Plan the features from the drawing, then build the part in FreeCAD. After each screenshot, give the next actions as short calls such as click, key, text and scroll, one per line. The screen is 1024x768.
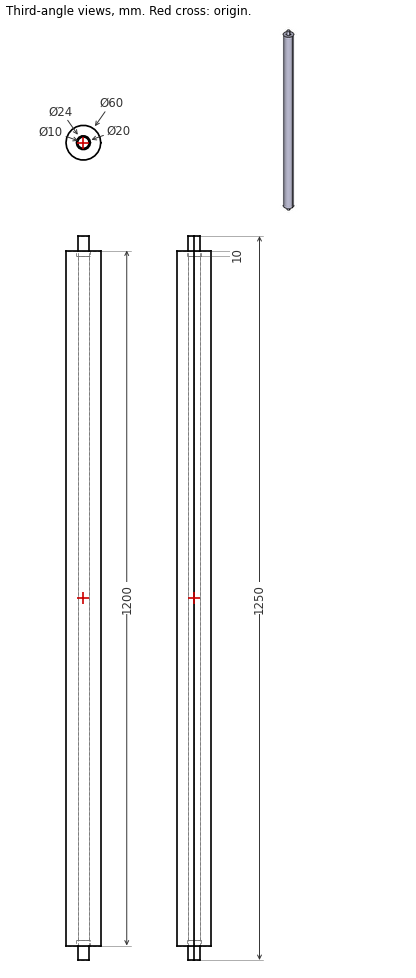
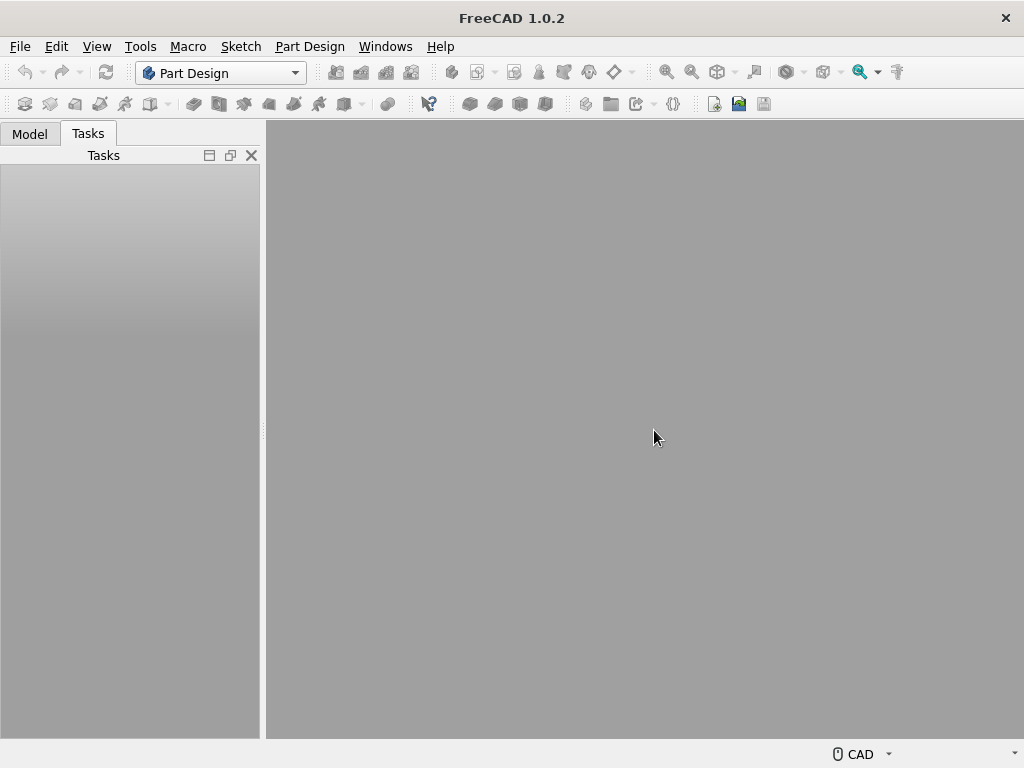
key(ctrl+n)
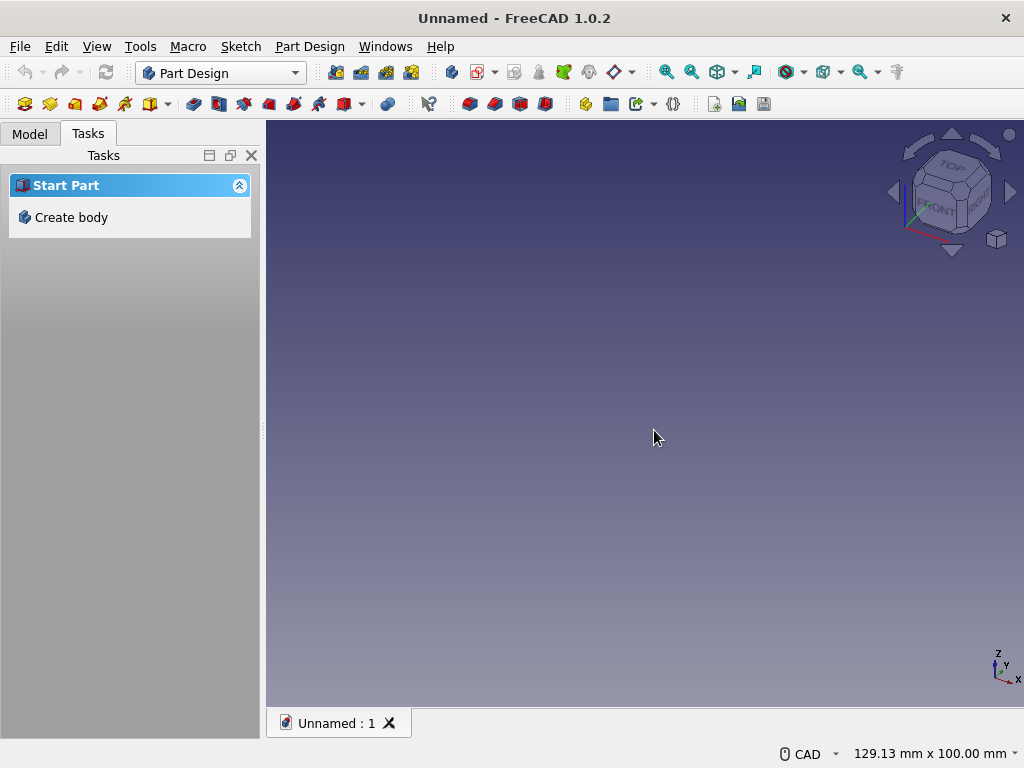
click(476, 72)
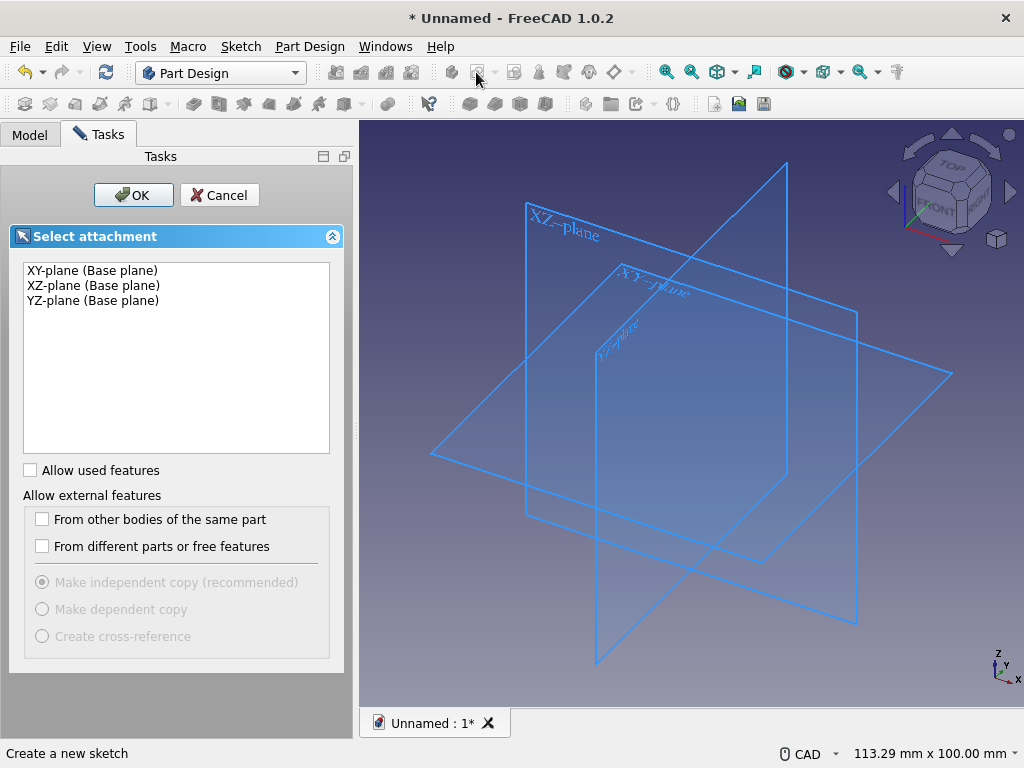
click(84, 270)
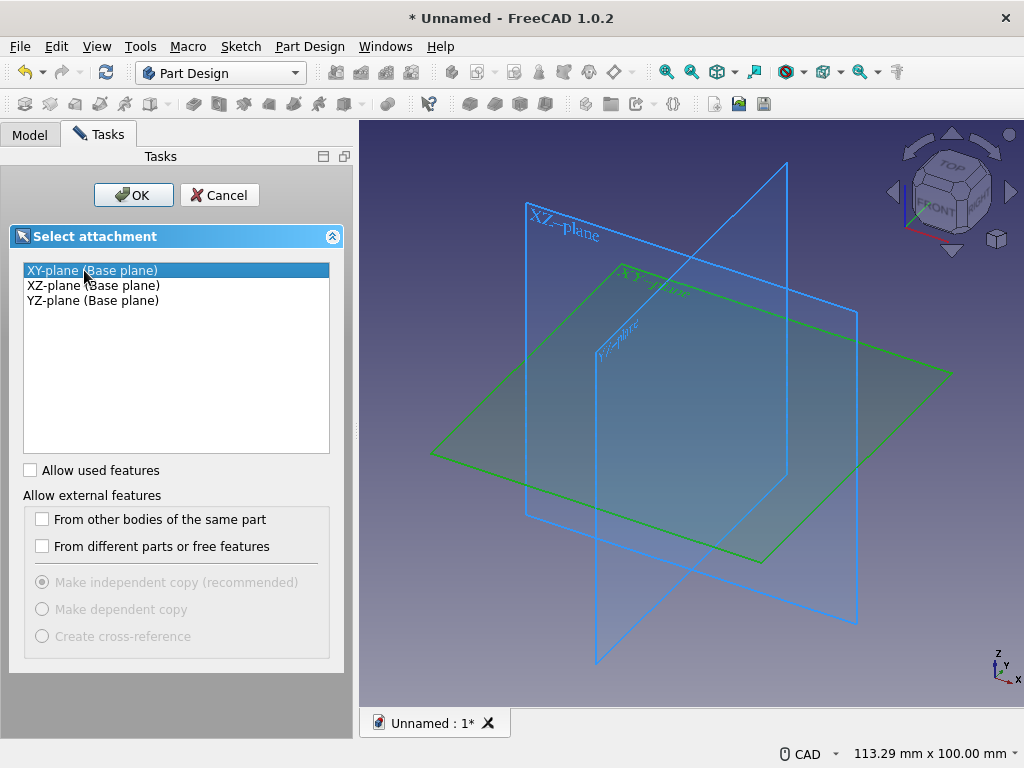
click(134, 195)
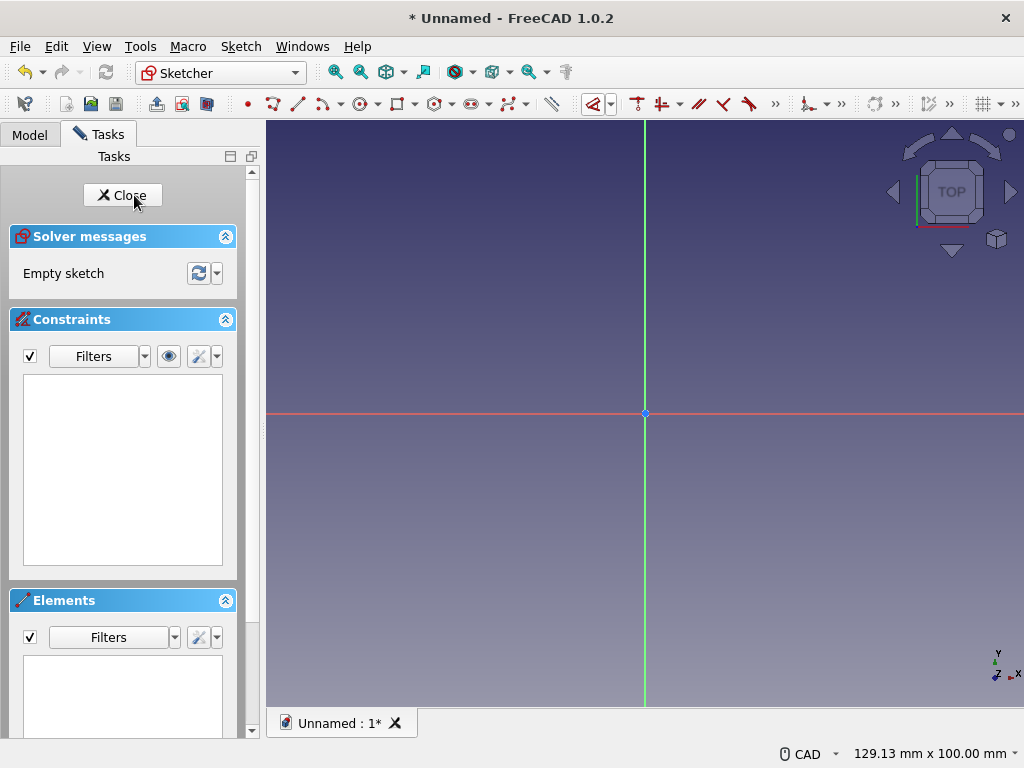
scroll(675, 414, up, 6)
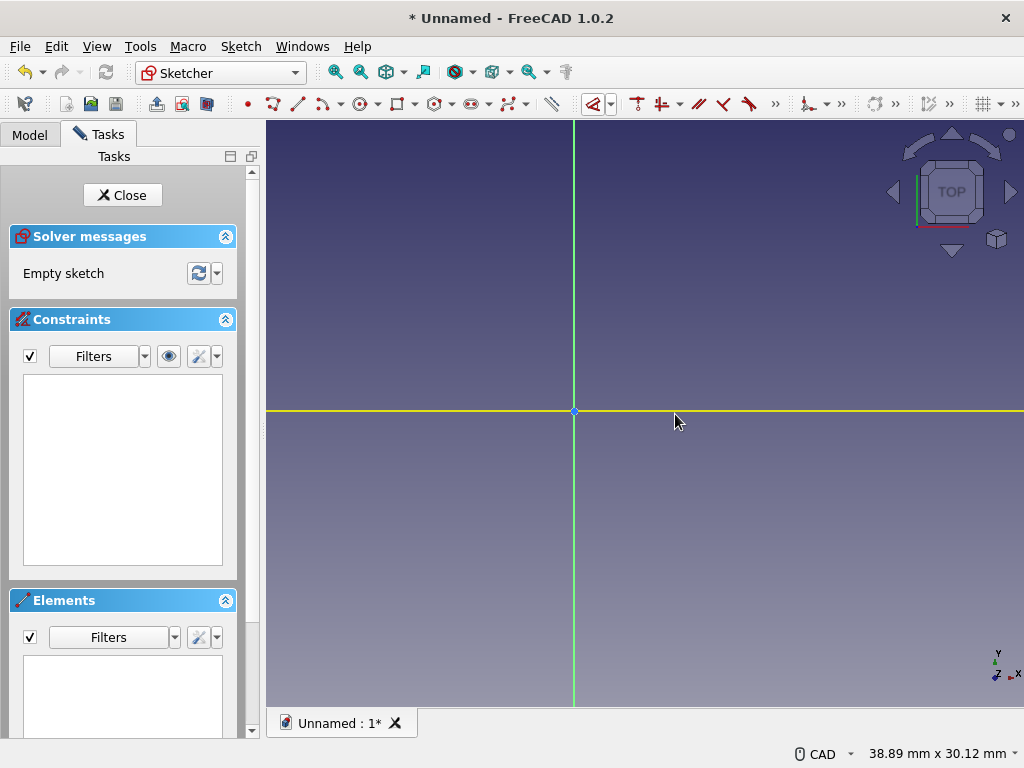
click(360, 104)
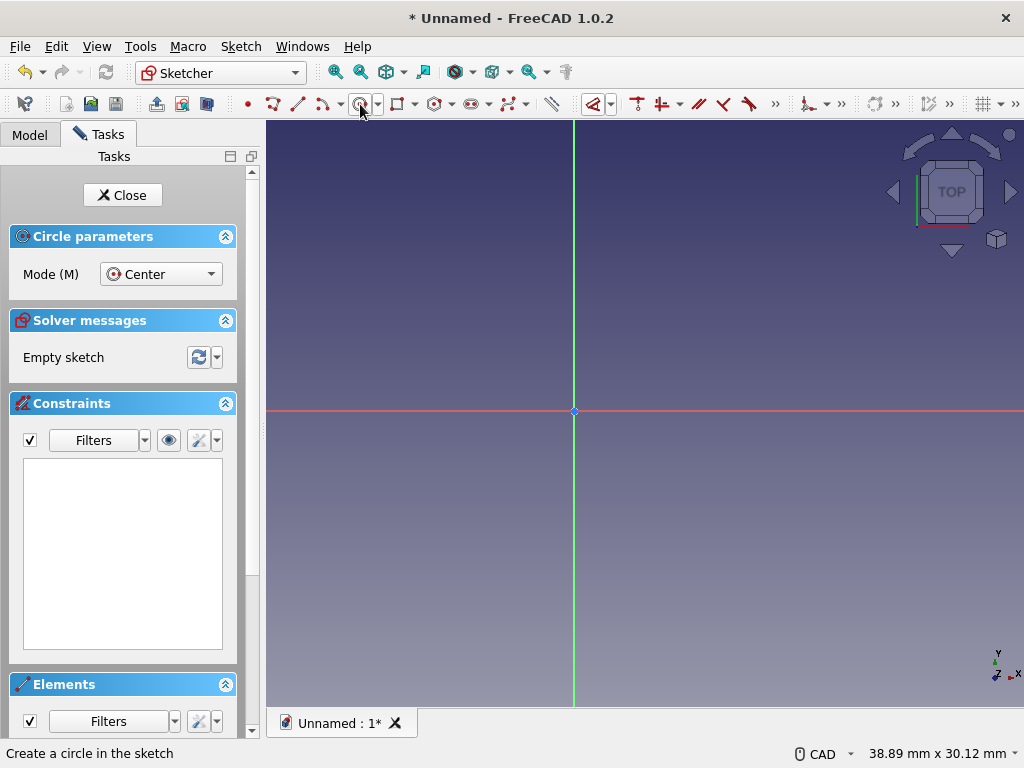
click(574, 411)
click(712, 273)
key(Escape)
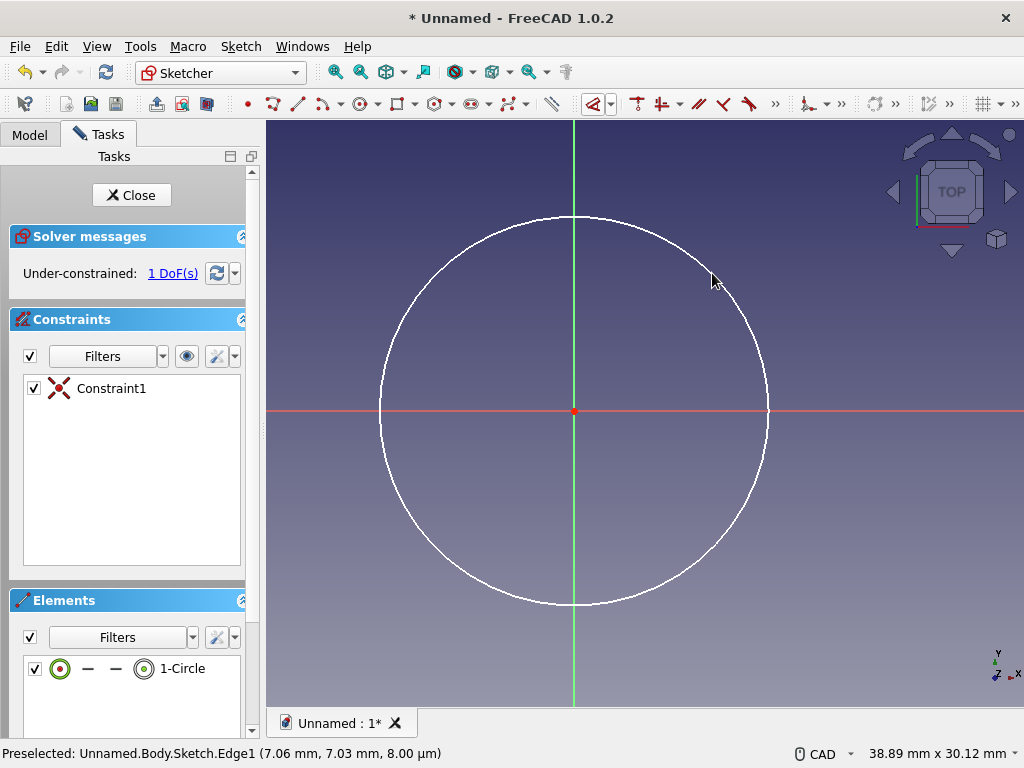
key(d)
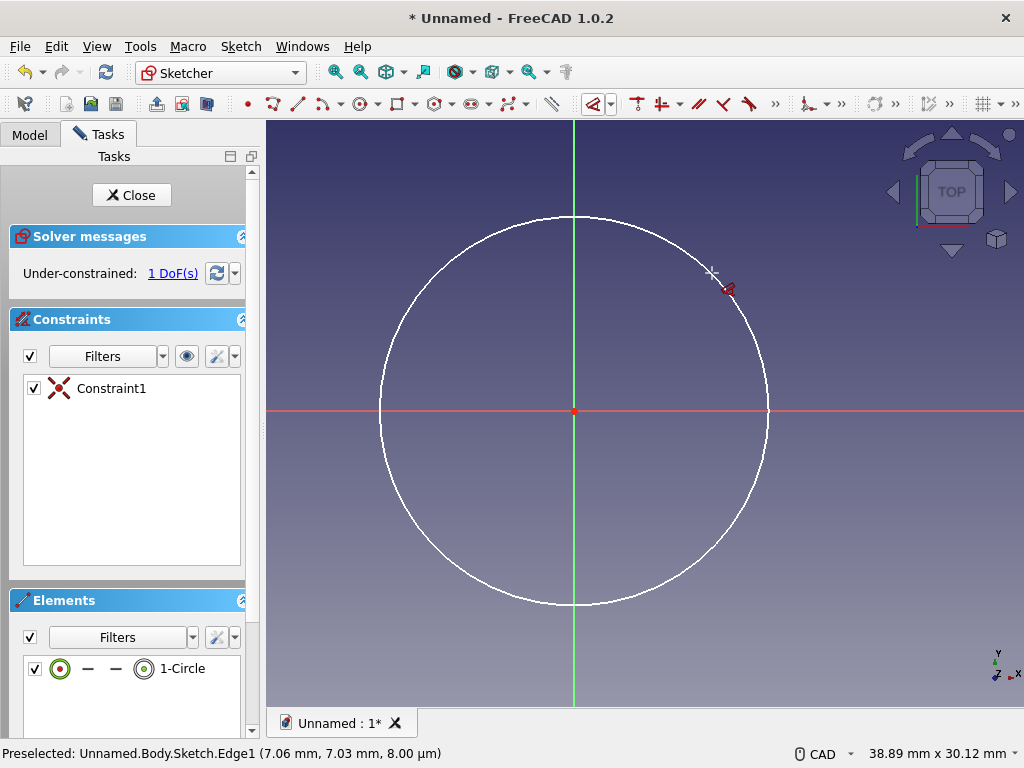
click(711, 273)
click(734, 250)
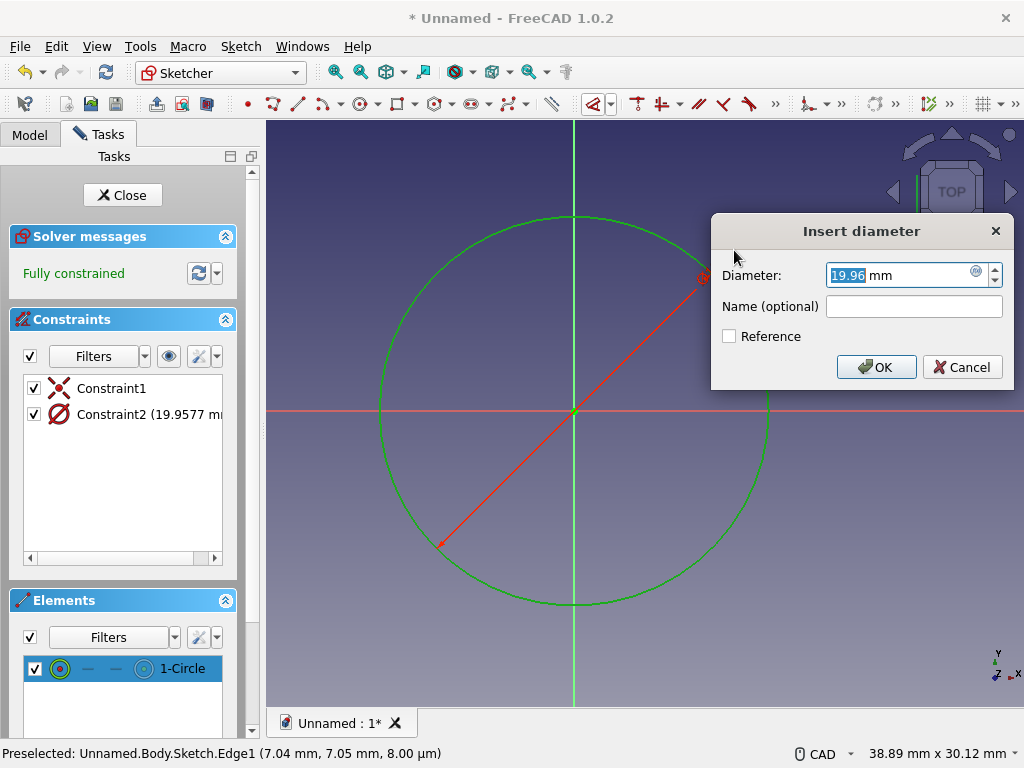
text(20)
key(Return)
key(Escape)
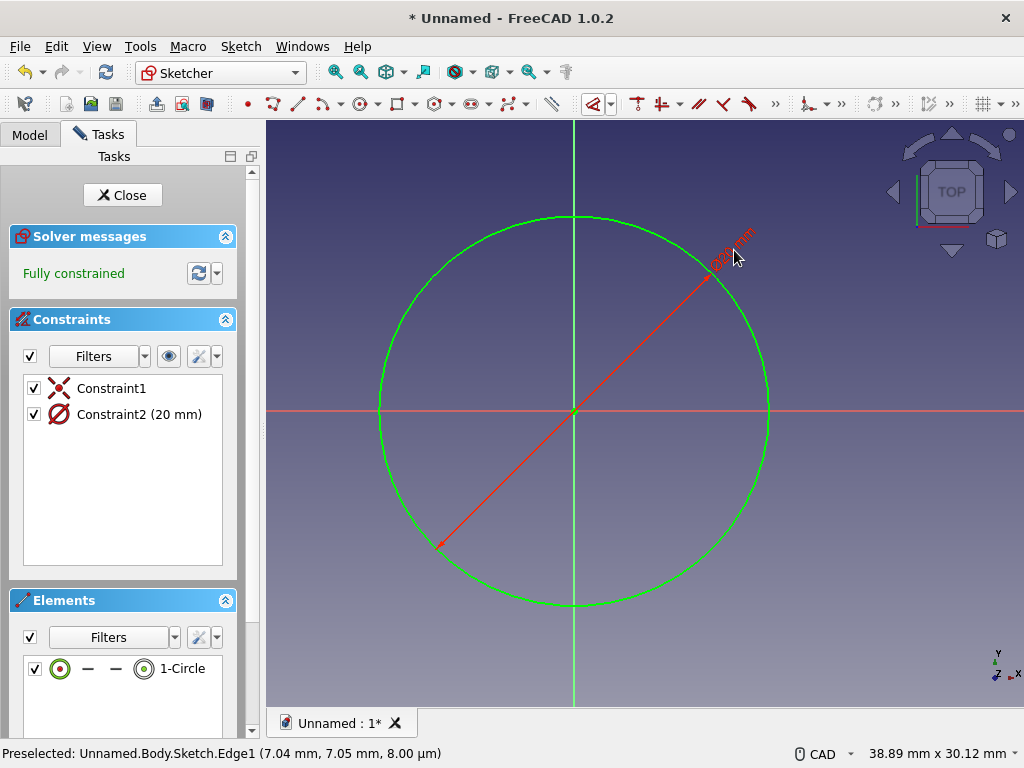
click(123, 195)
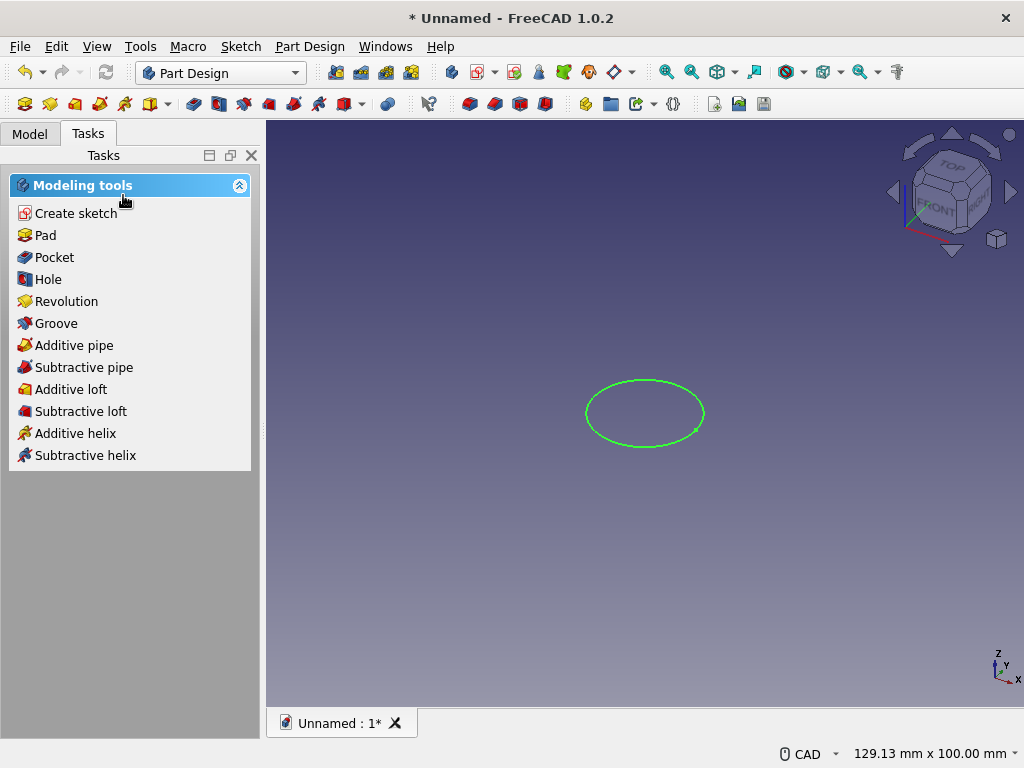
click(25, 104)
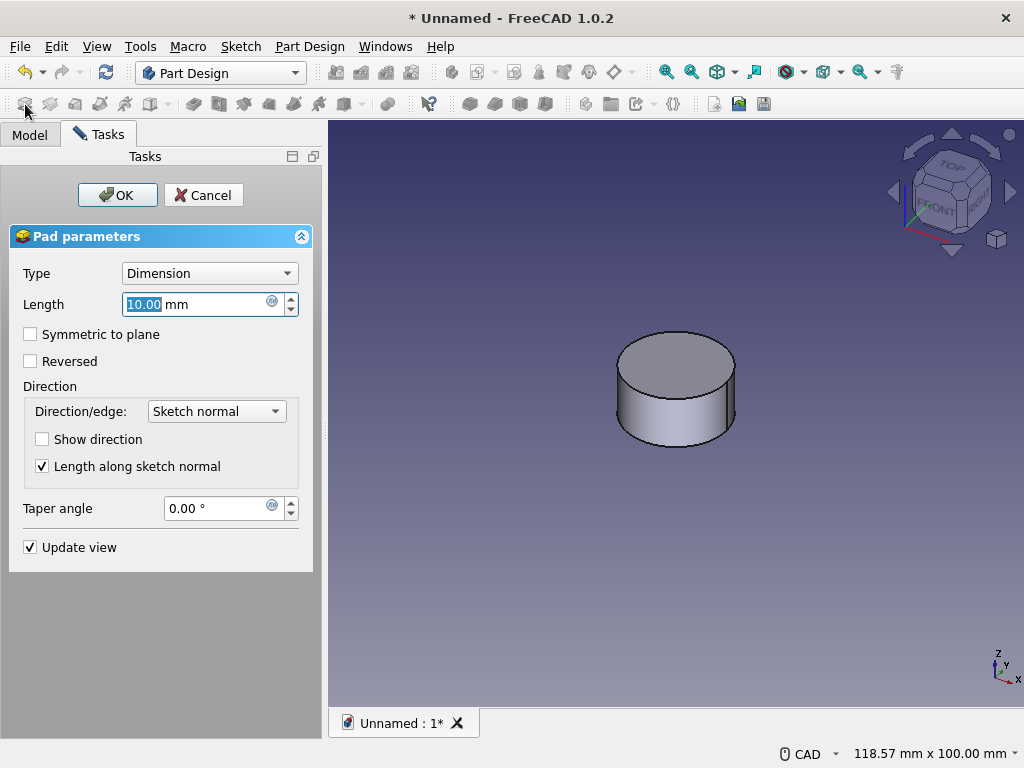
text(1250)
key(Tab)